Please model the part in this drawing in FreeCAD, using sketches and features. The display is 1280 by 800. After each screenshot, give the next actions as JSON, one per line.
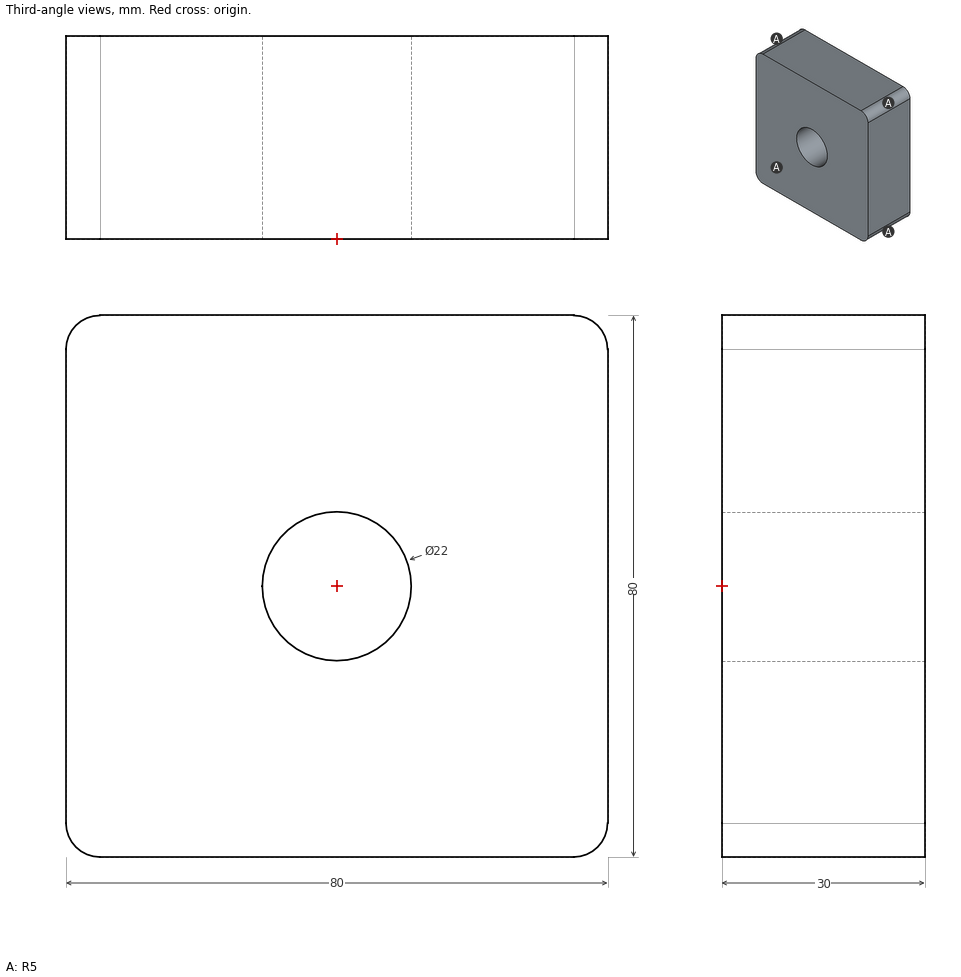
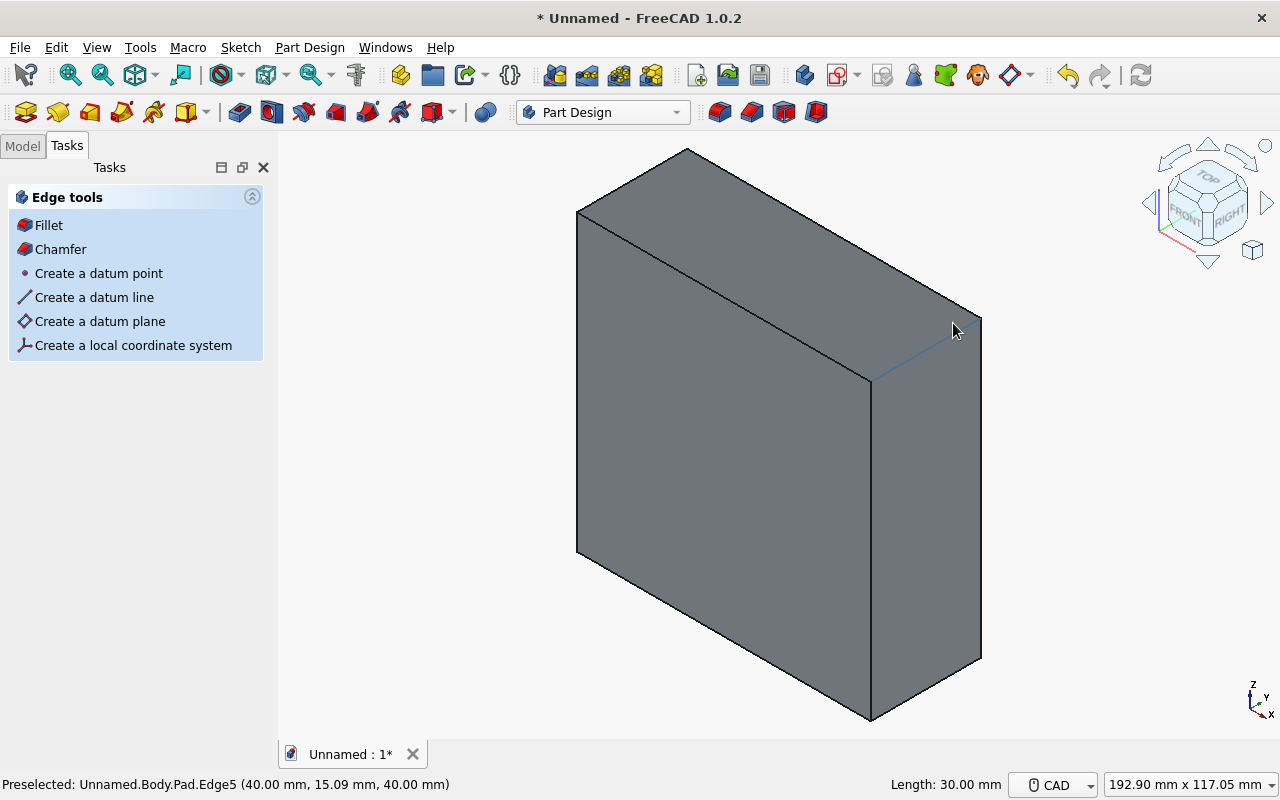
{"action": "key", "text": "2"}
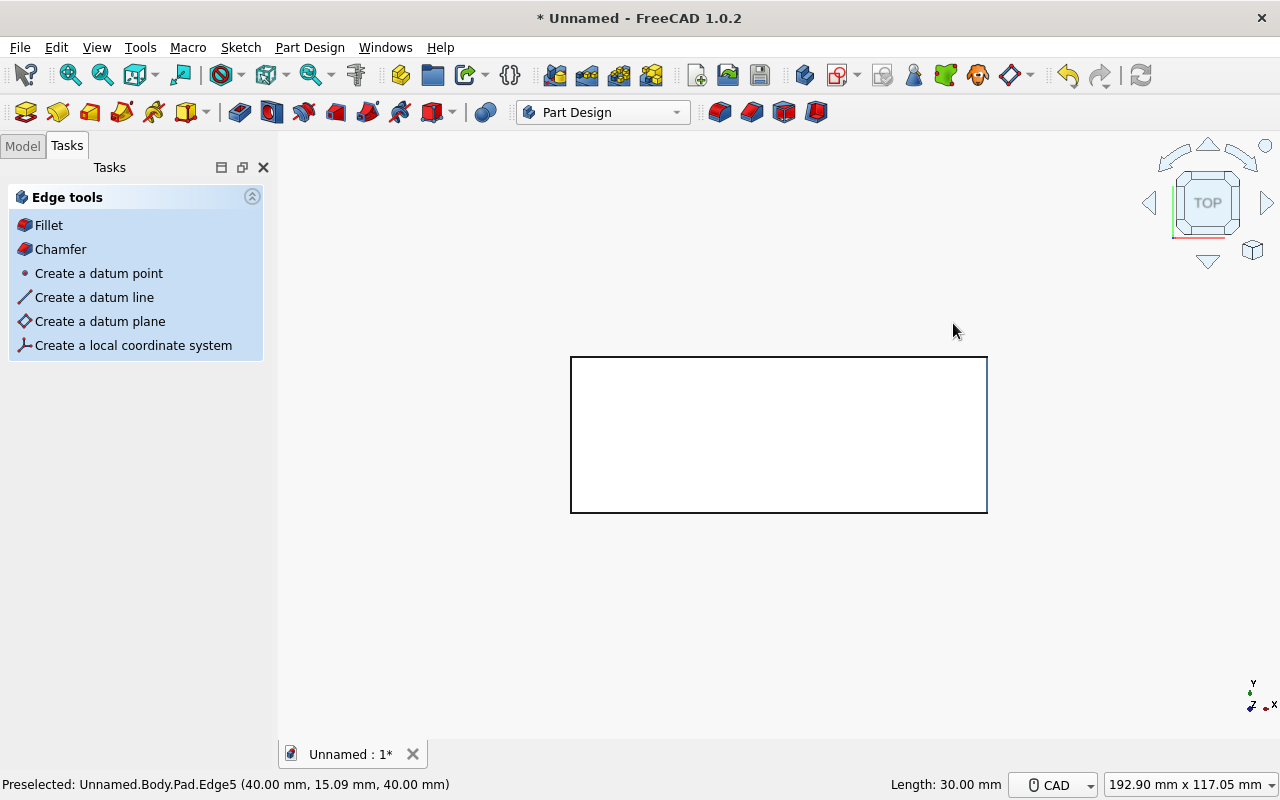
{"action": "left_click", "coordinate": [72, 76]}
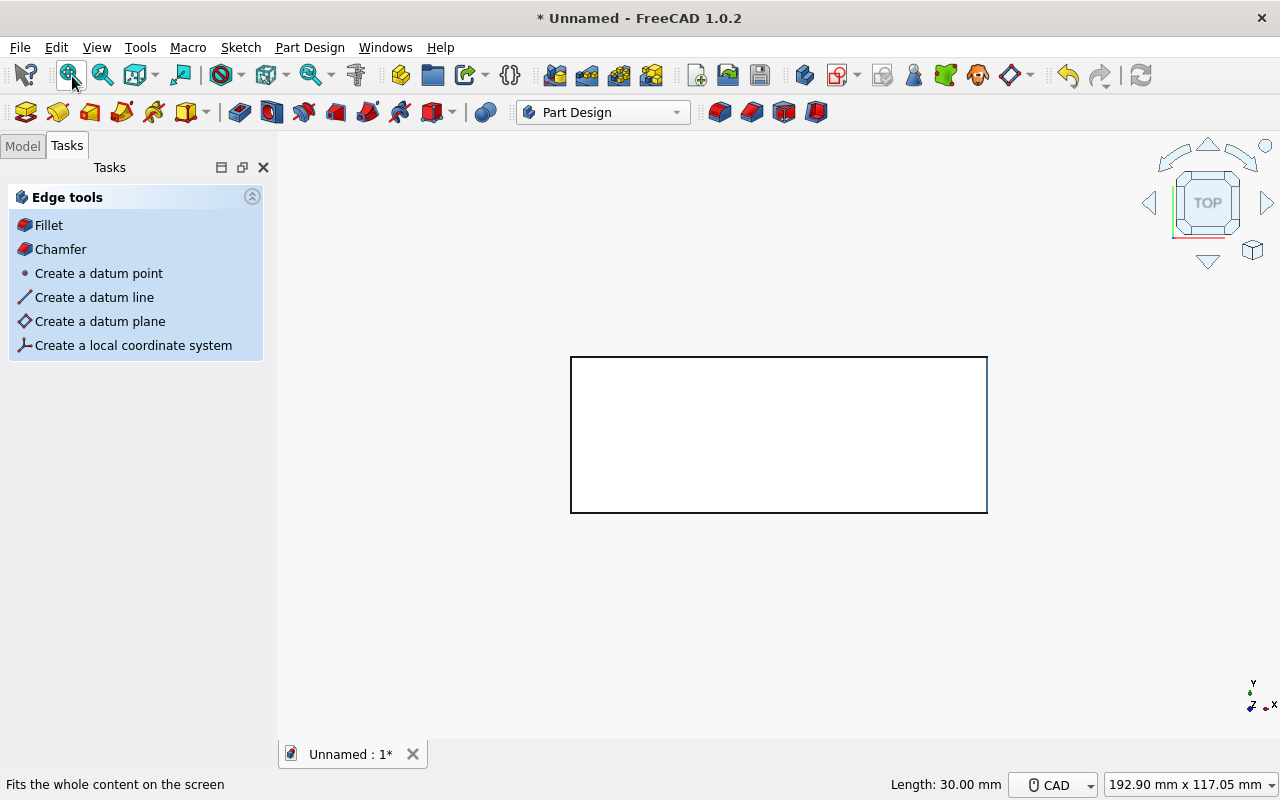
{"action": "left_click", "coordinate": [571, 434], "text": "ctrl"}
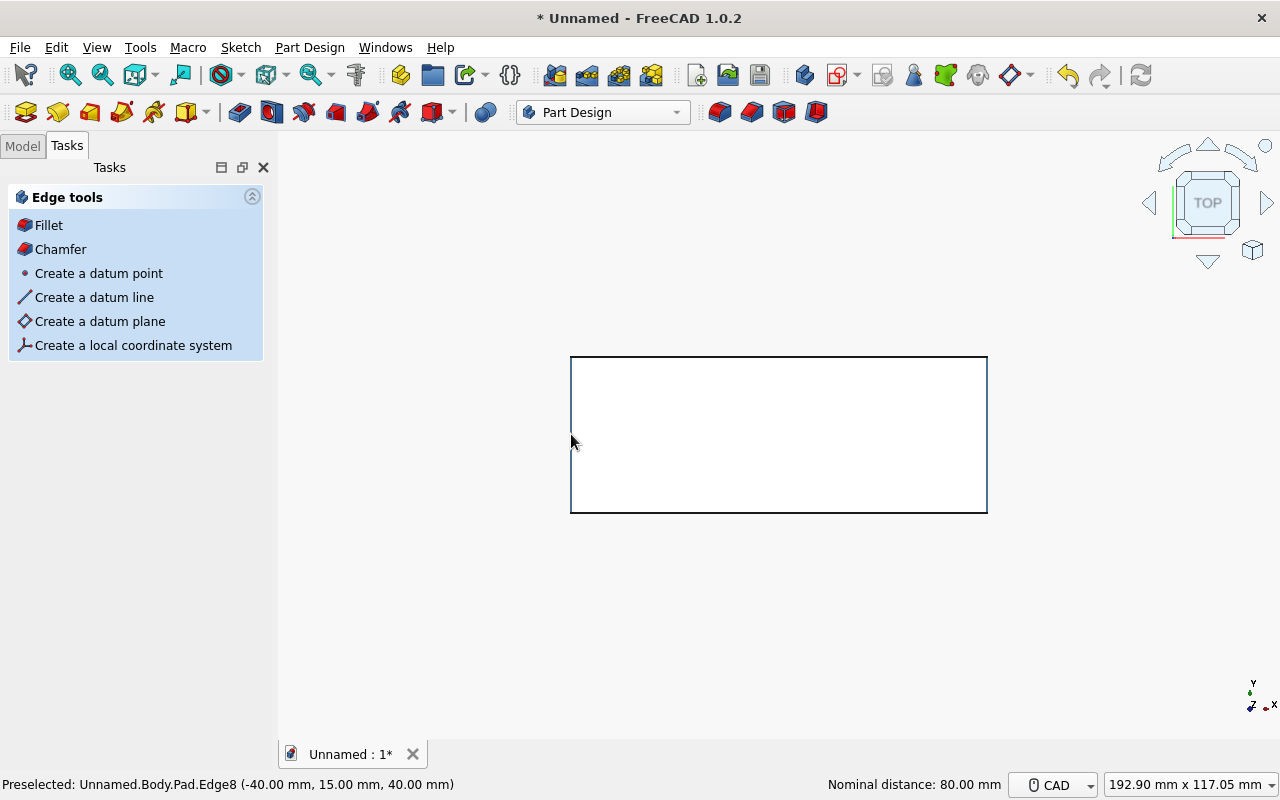
{"action": "key", "text": "1"}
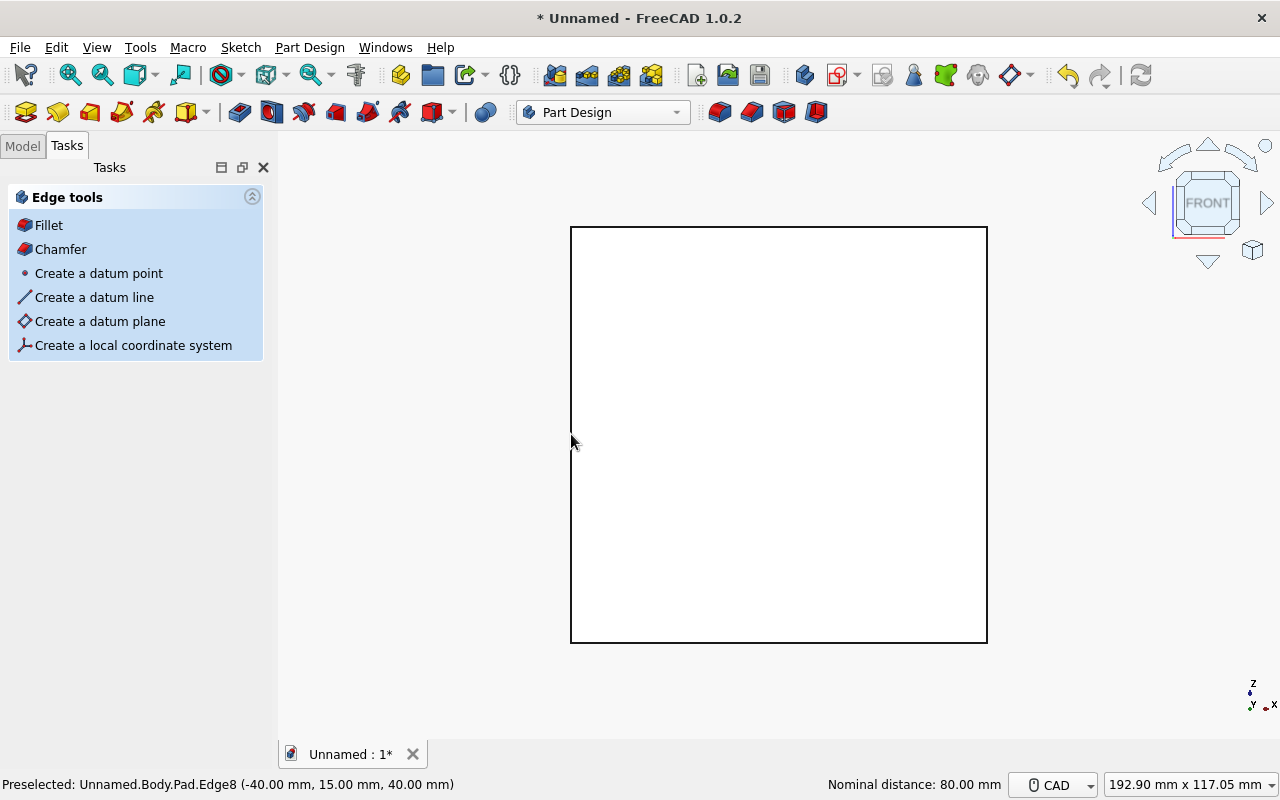
{"action": "key", "text": "3"}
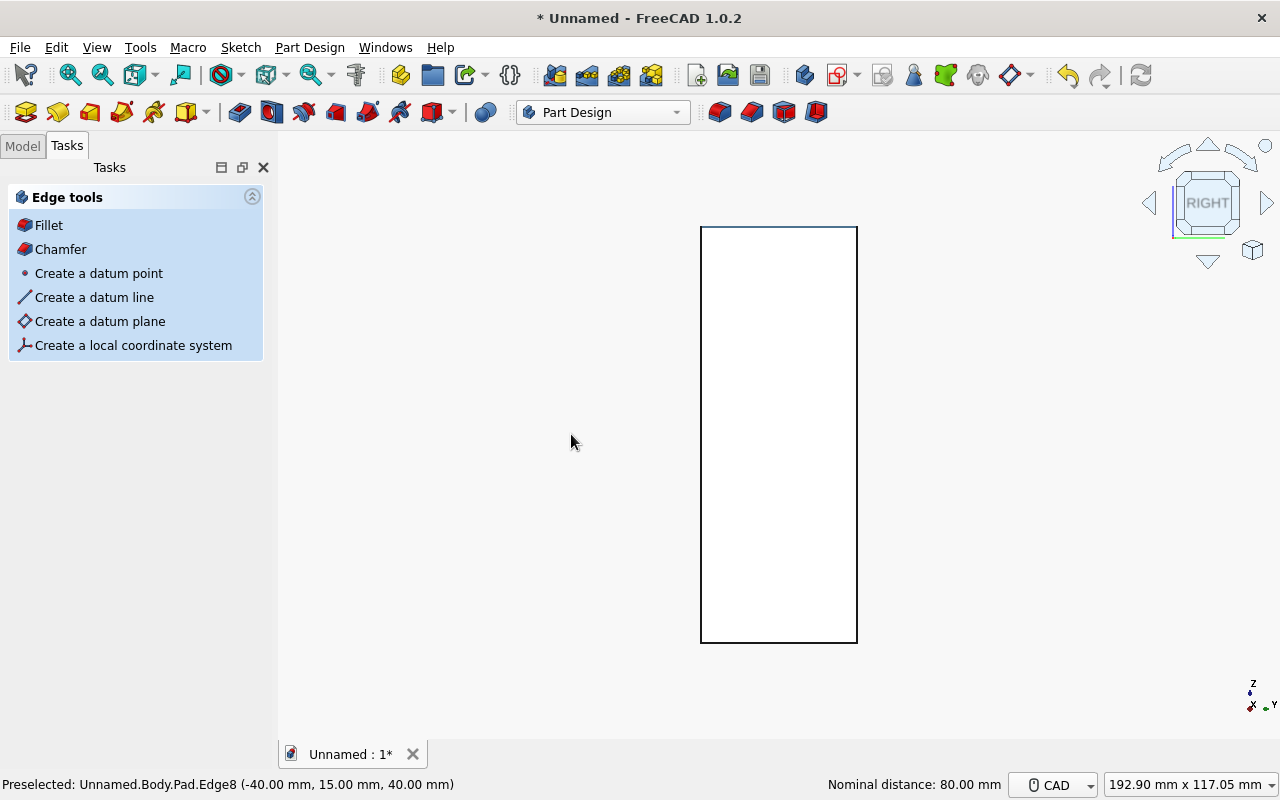
{"action": "left_click", "coordinate": [779, 642], "text": "ctrl"}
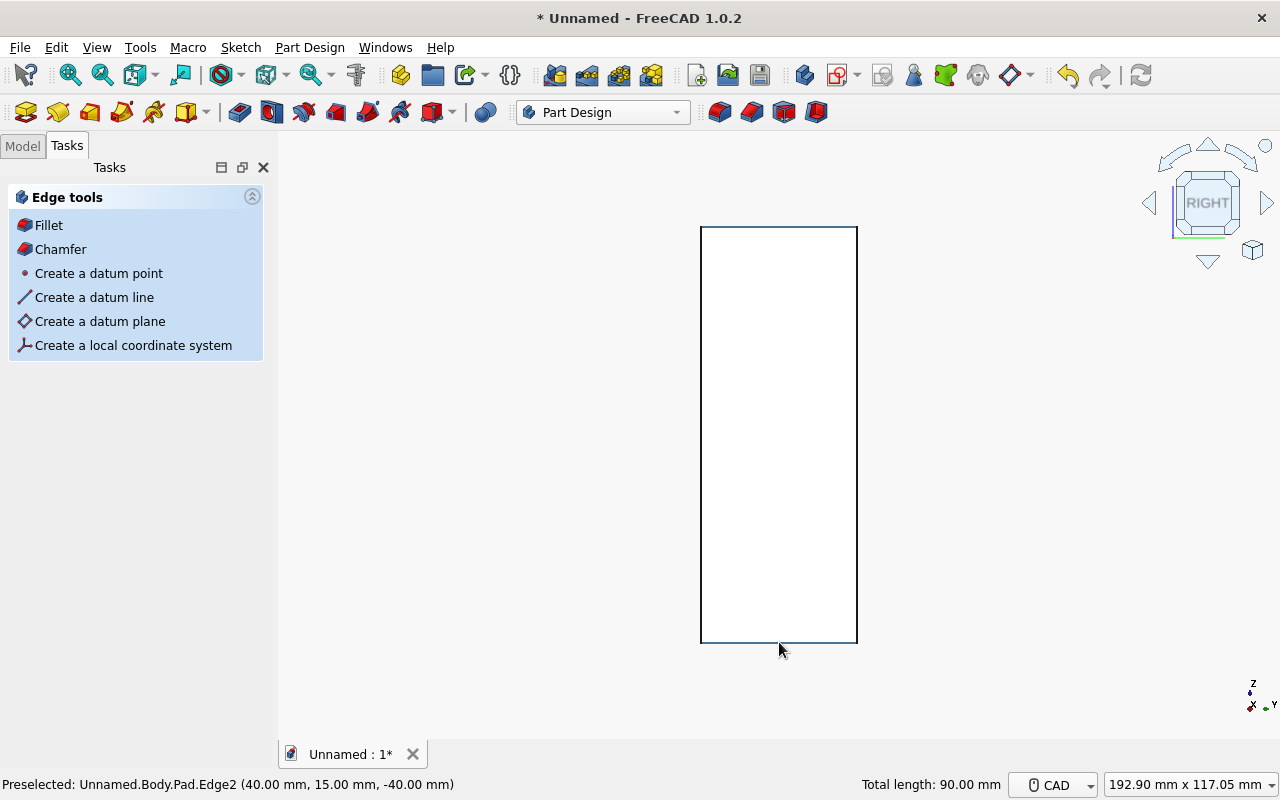
{"action": "key", "text": "5"}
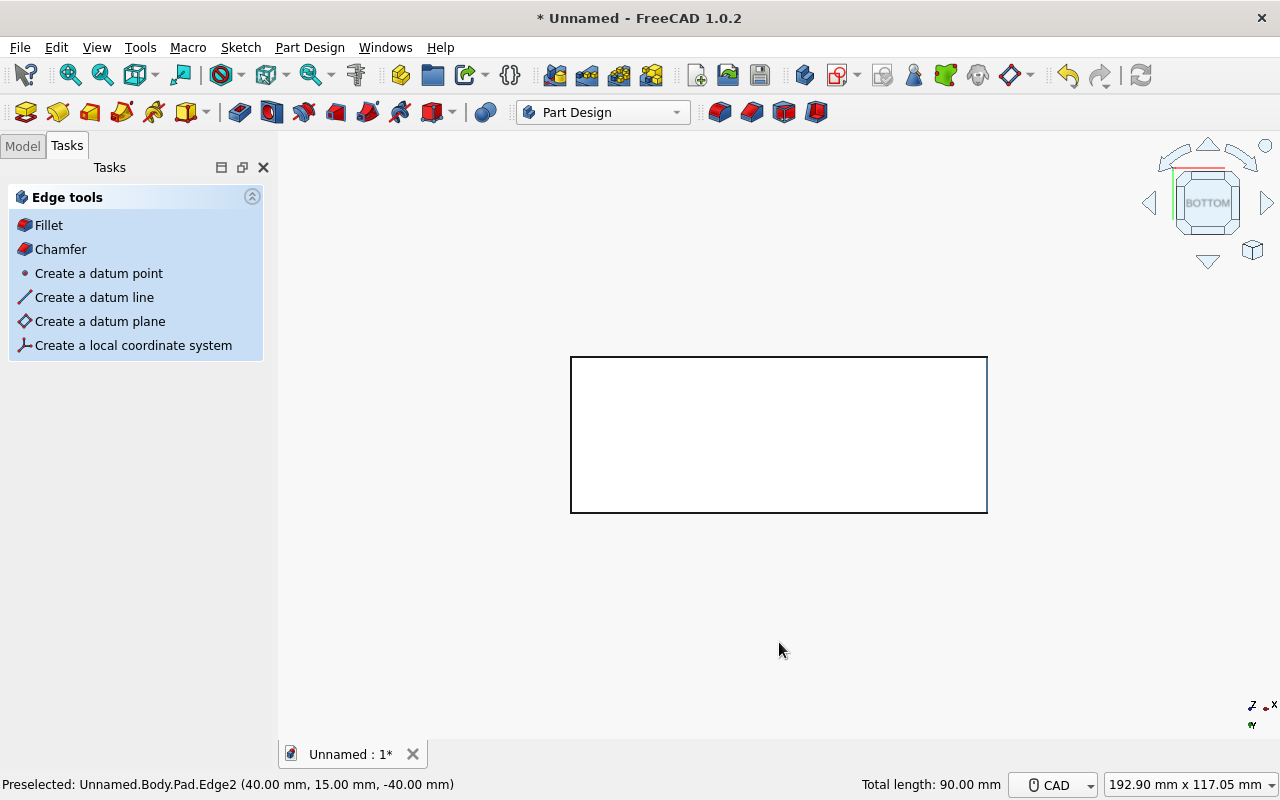
{"action": "left_click", "coordinate": [72, 76]}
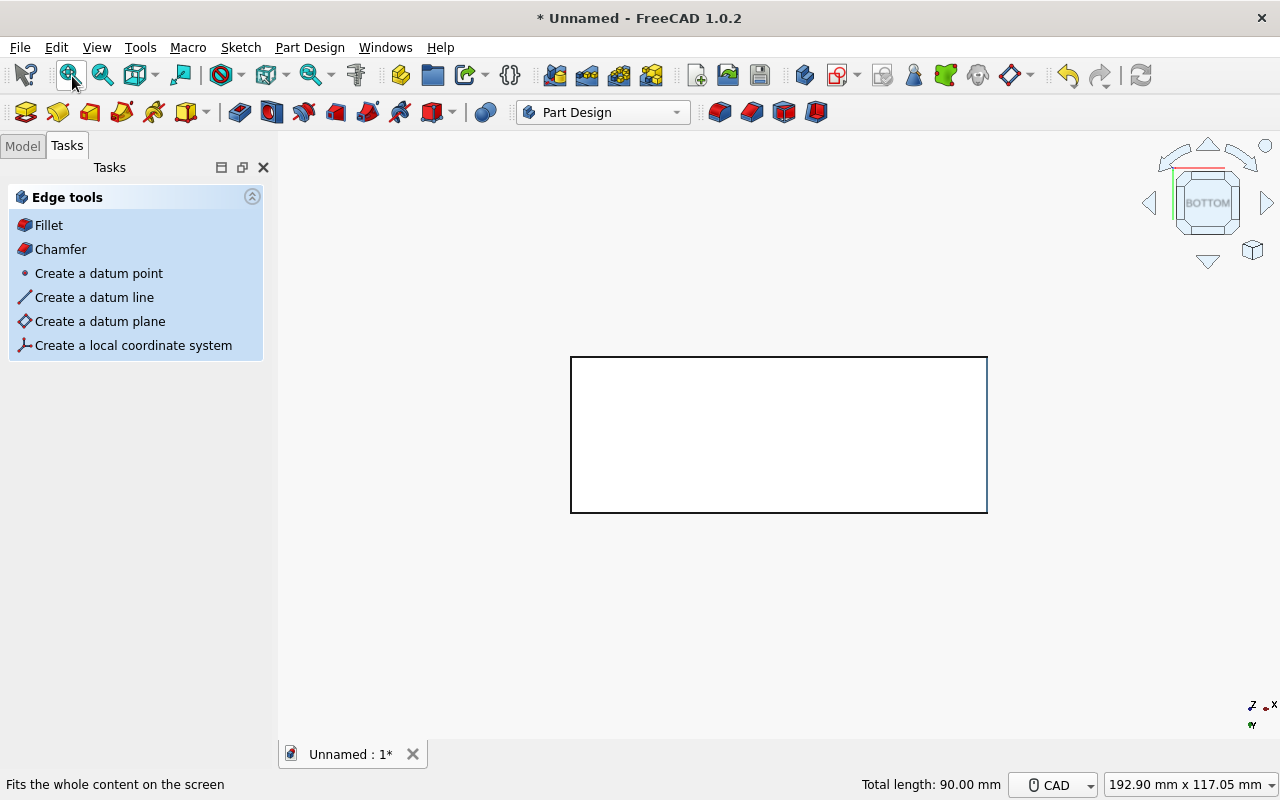
{"action": "left_click", "coordinate": [571, 434], "text": "ctrl"}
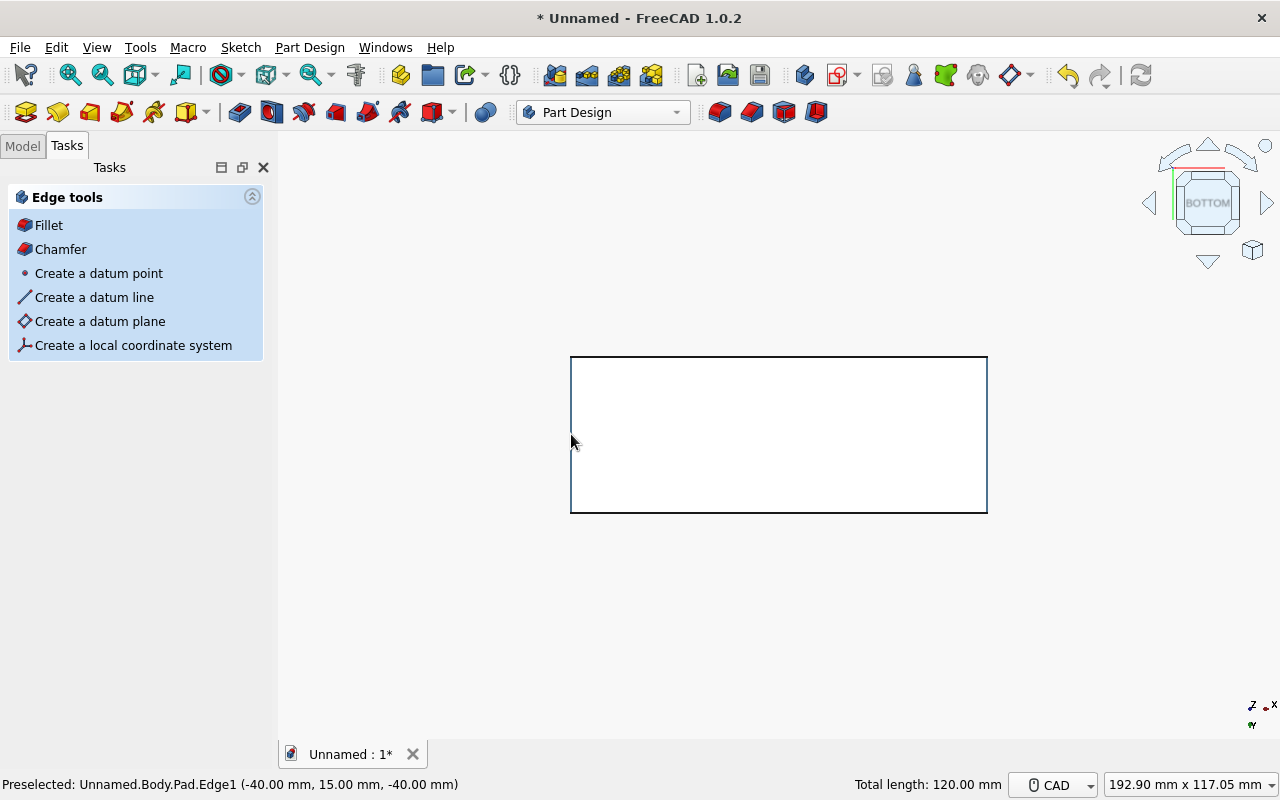
{"action": "left_click", "coordinate": [720, 112]}